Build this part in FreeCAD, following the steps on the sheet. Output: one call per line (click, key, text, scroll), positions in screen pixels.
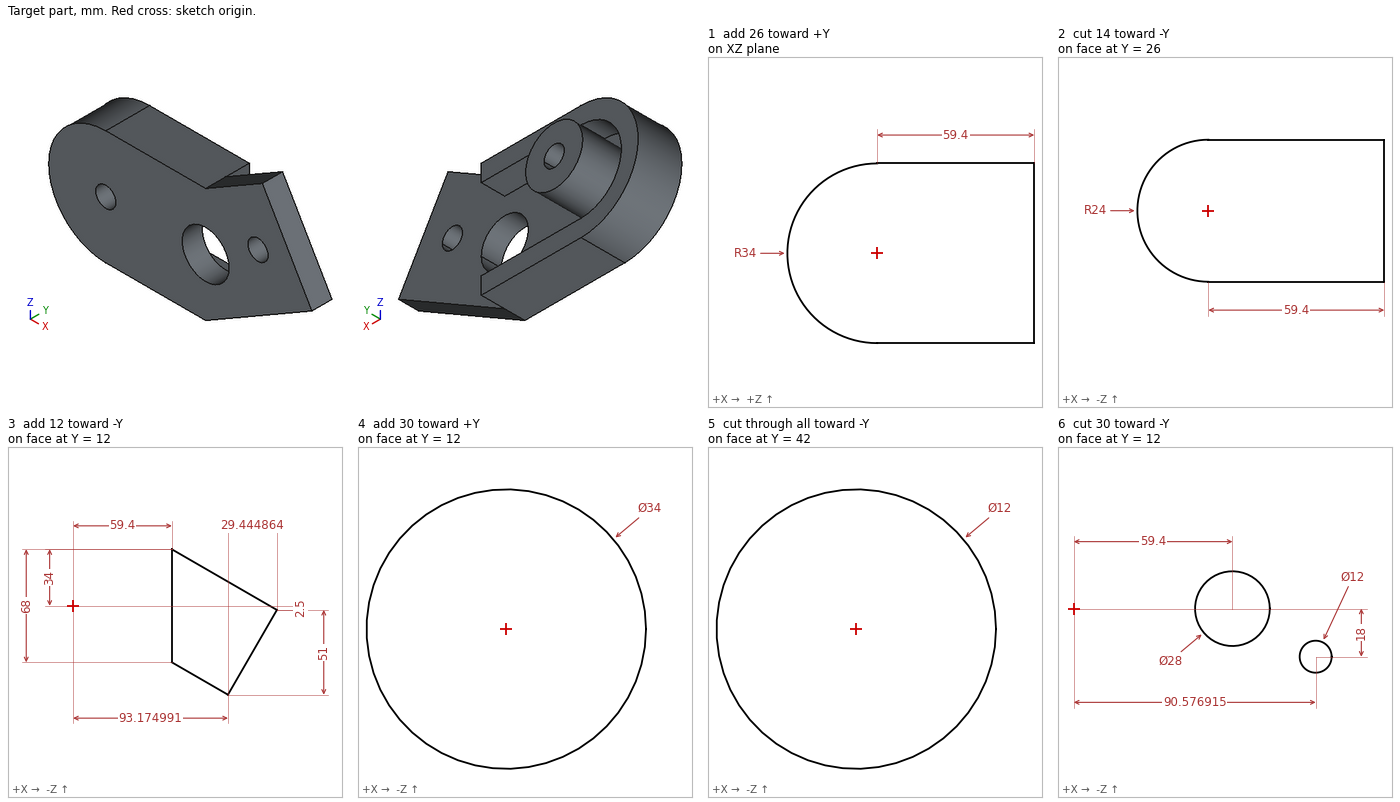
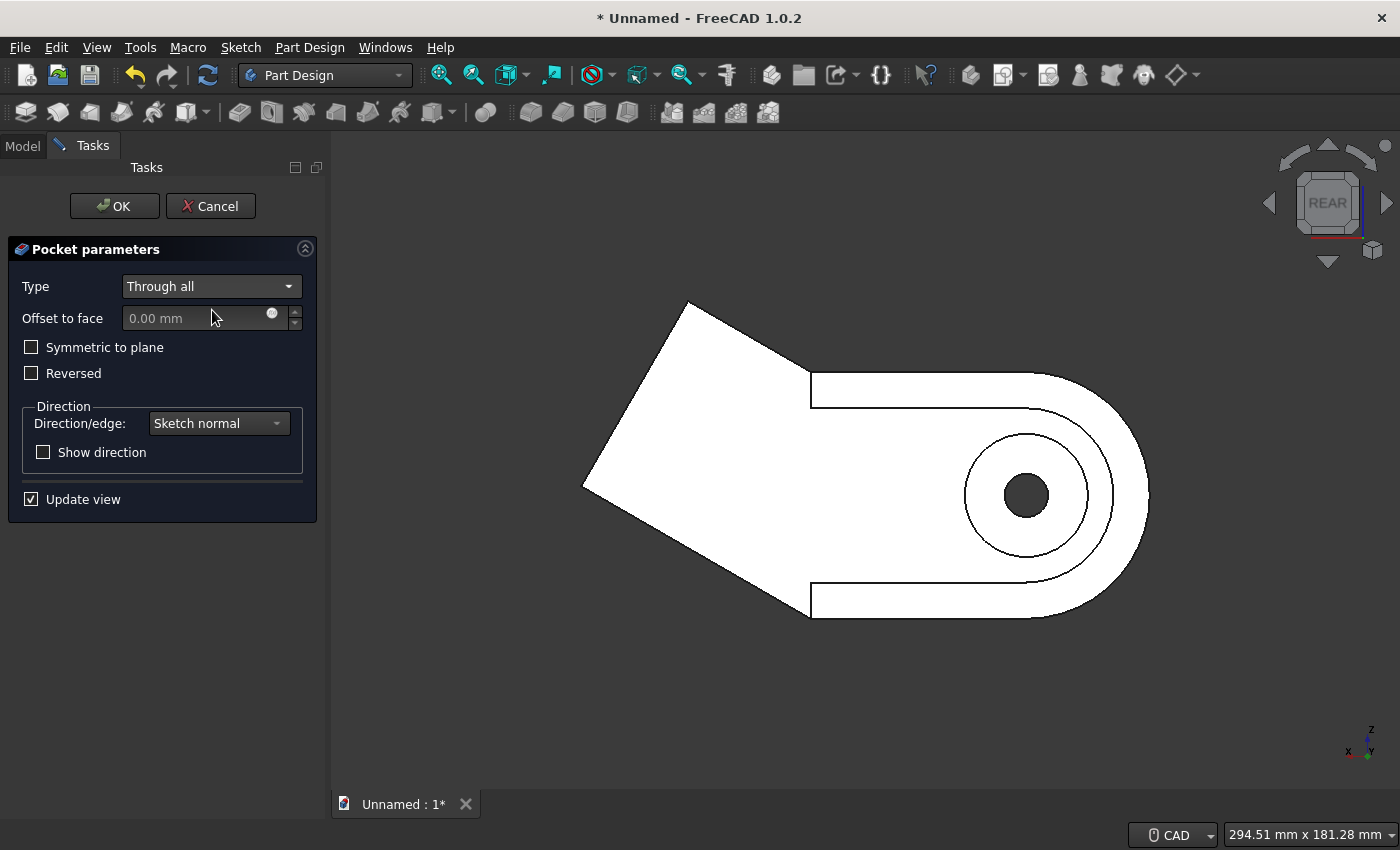
click(115, 206)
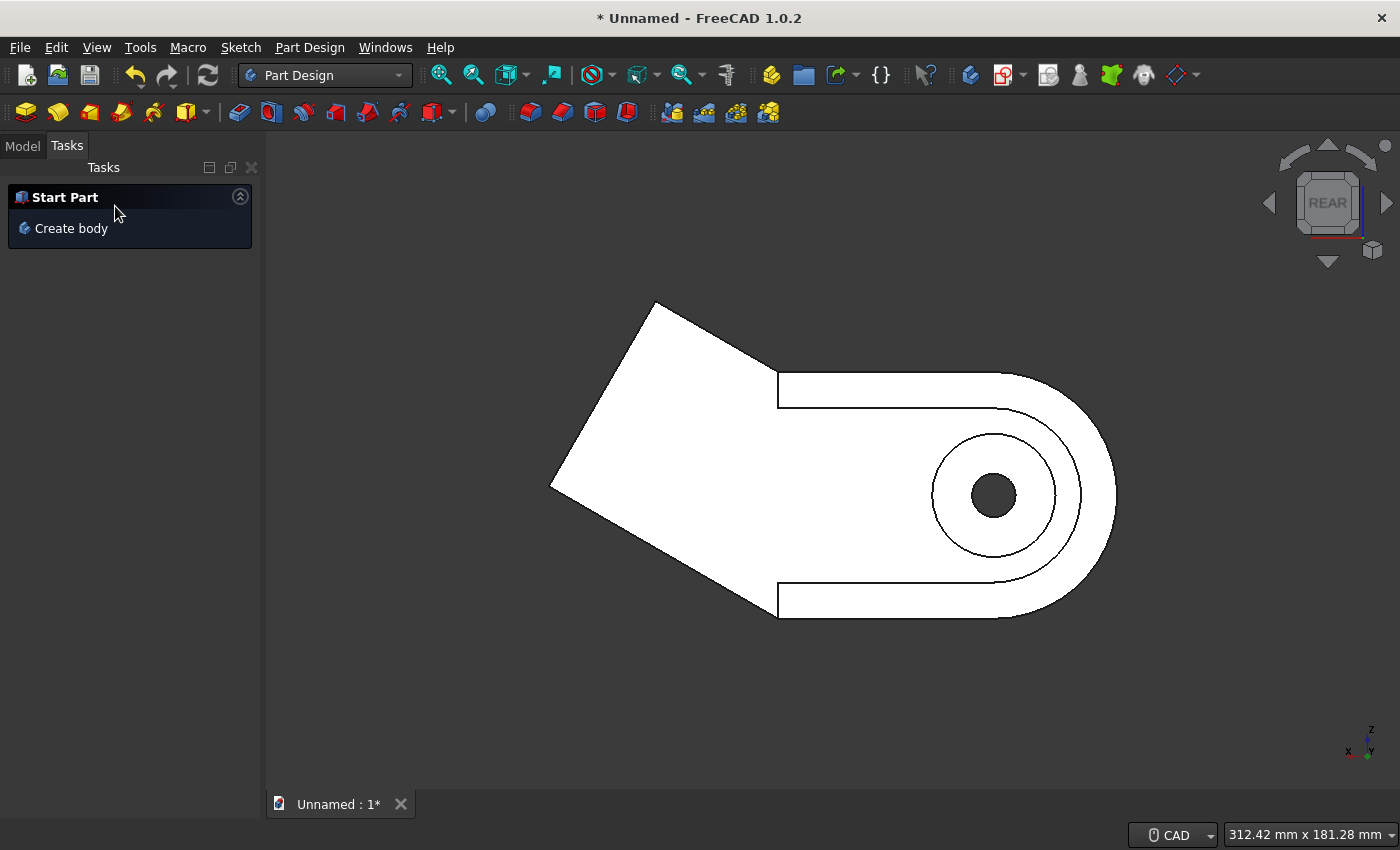
click(663, 459)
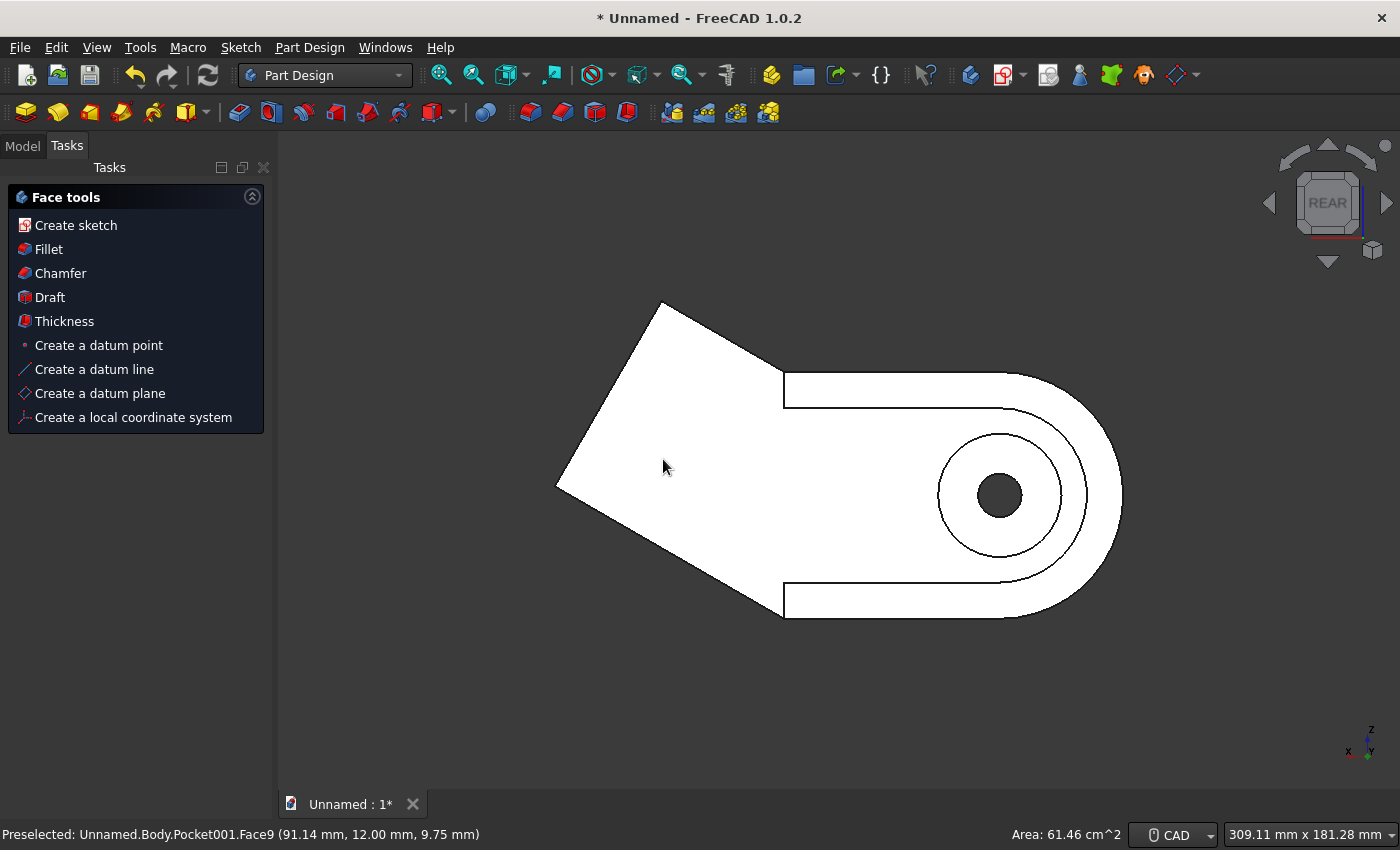
click(1004, 76)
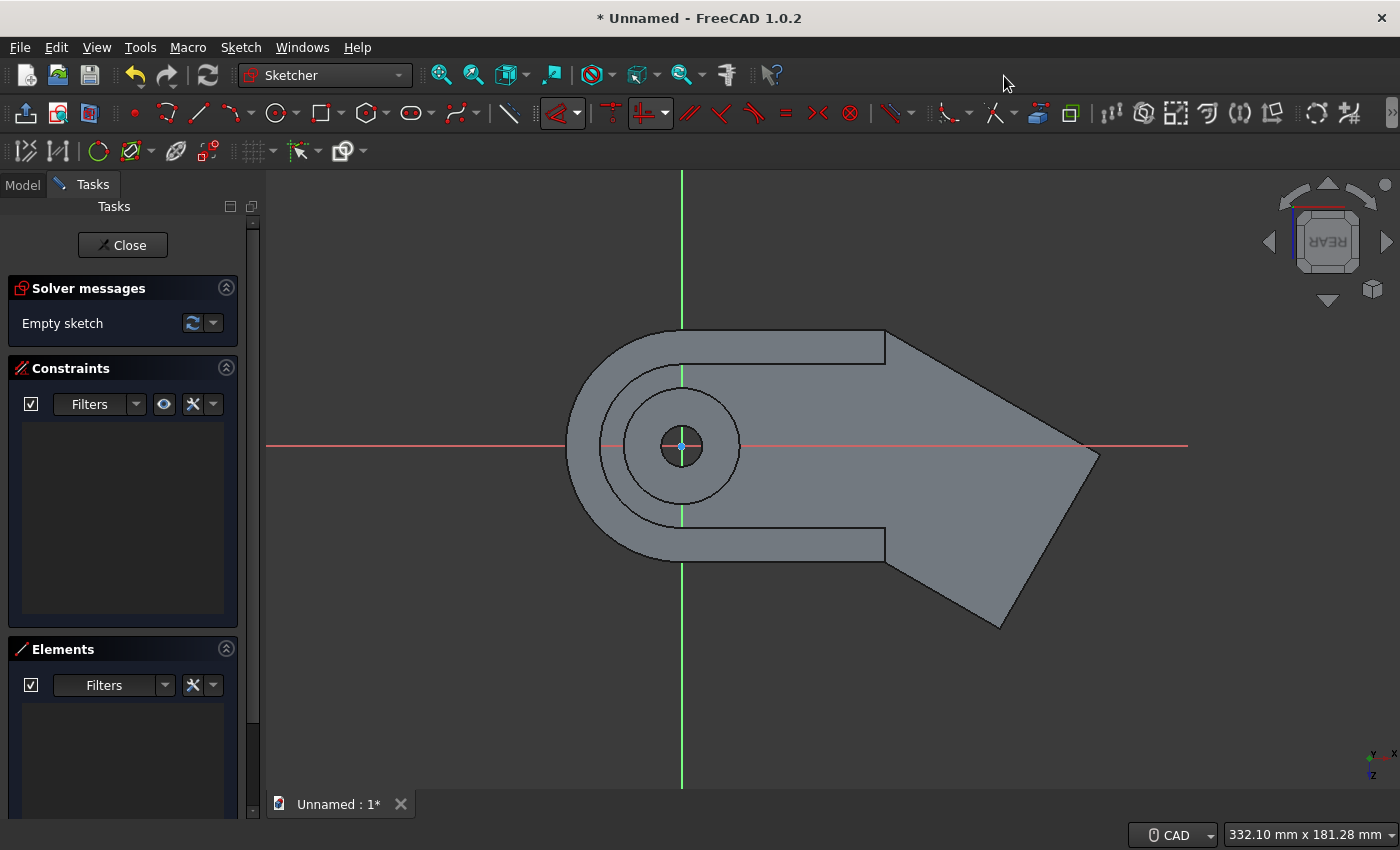
click(90, 114)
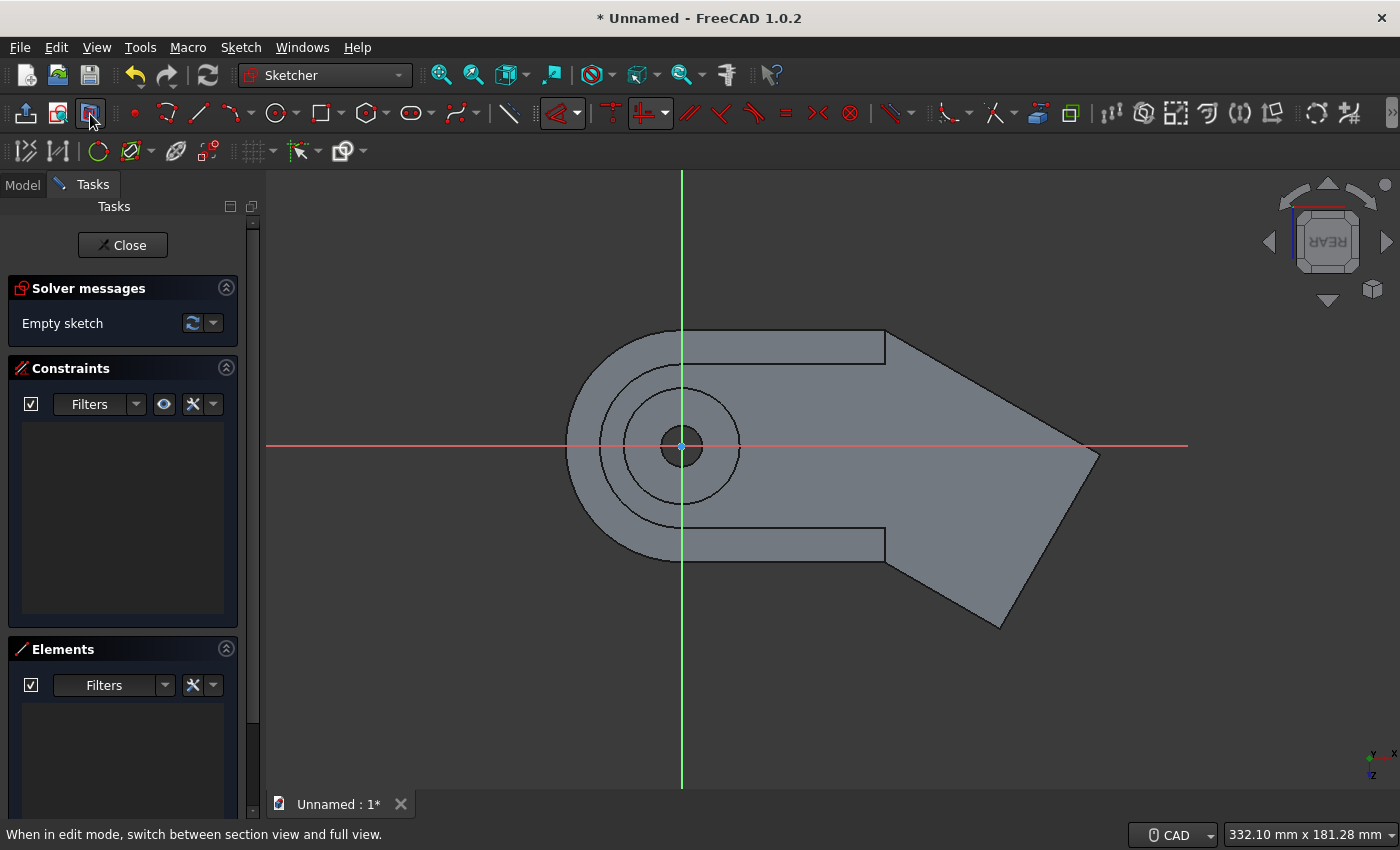
scroll(914, 450, up, 4)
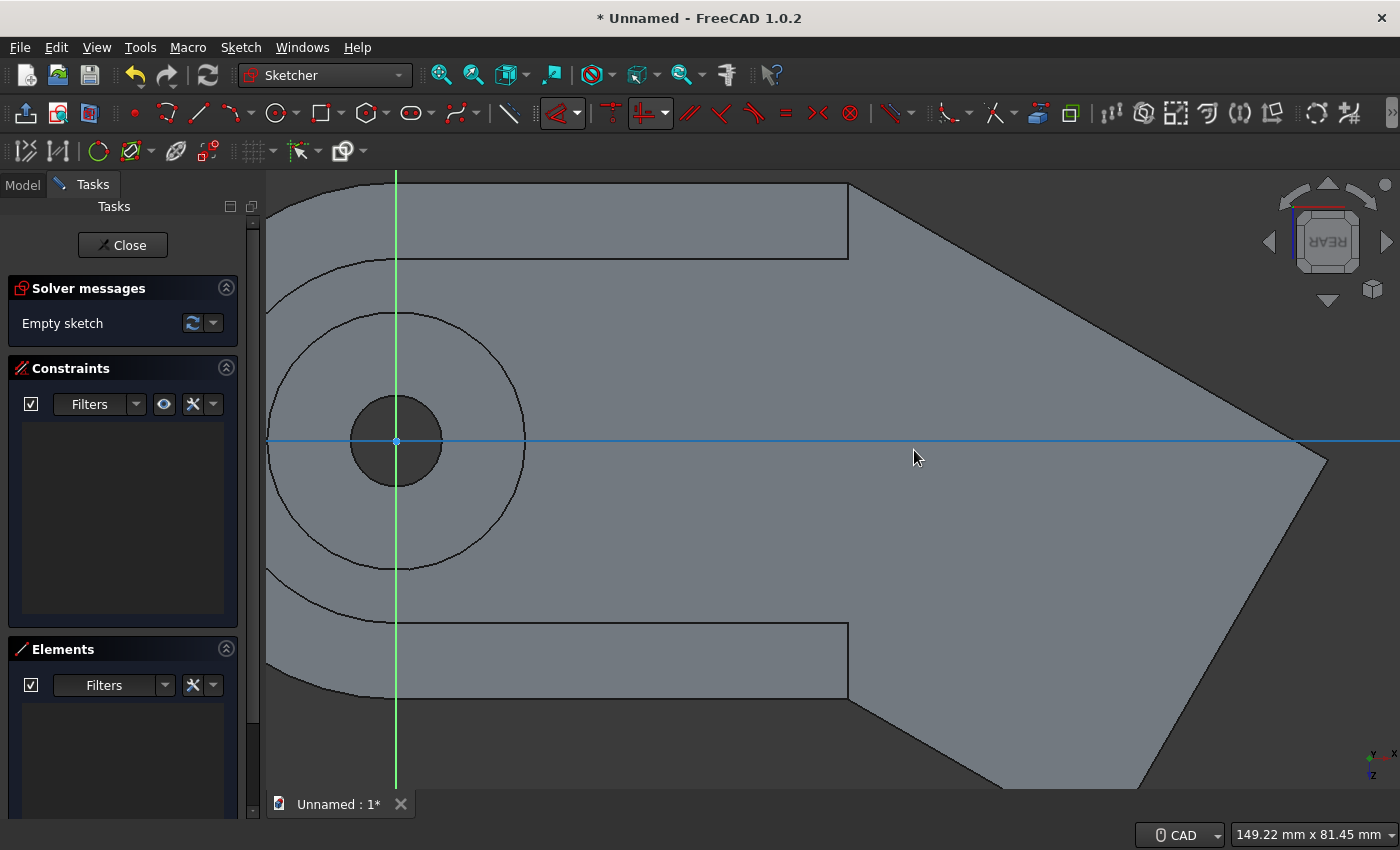
click(276, 114)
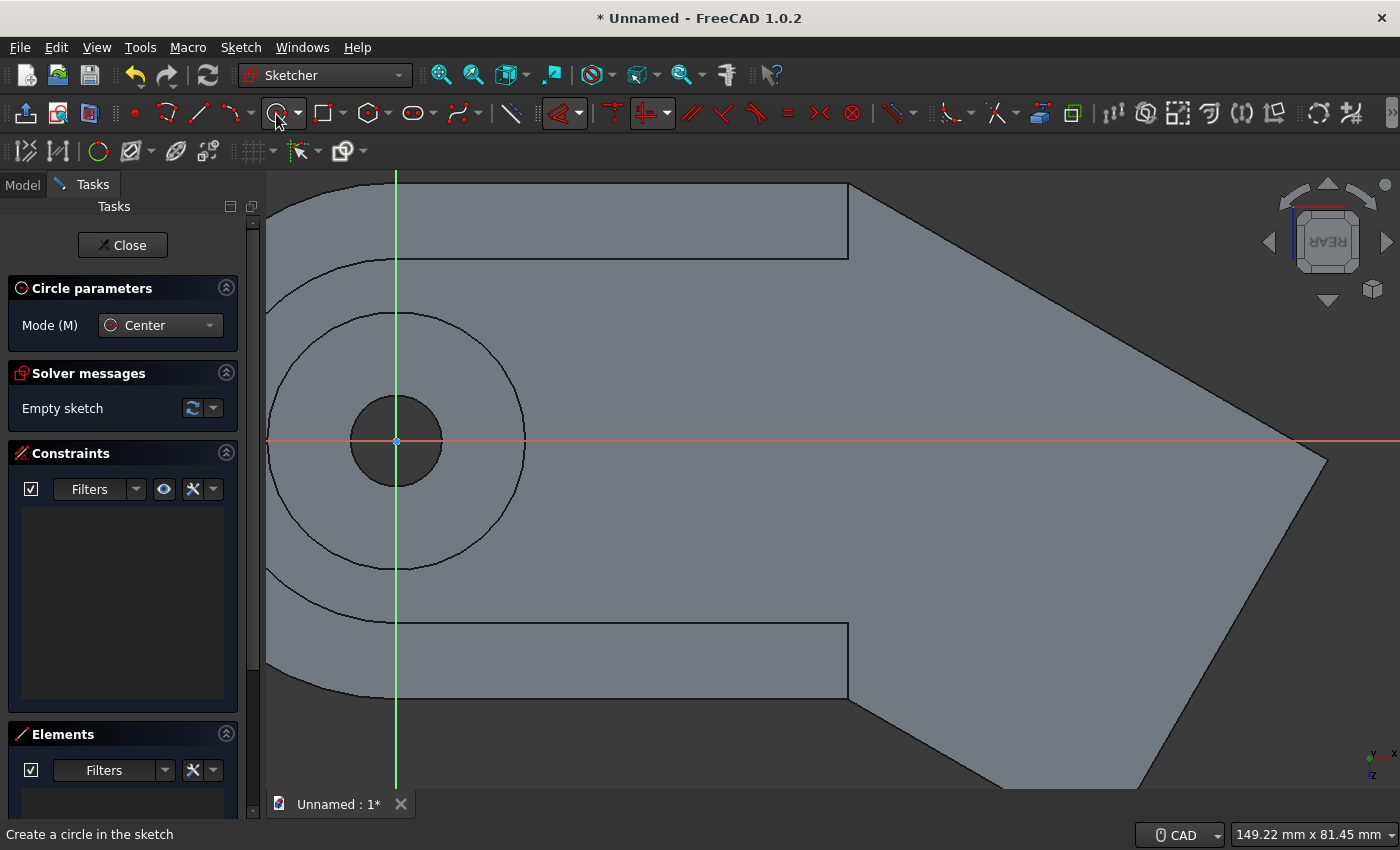
click(848, 441)
move(923, 366)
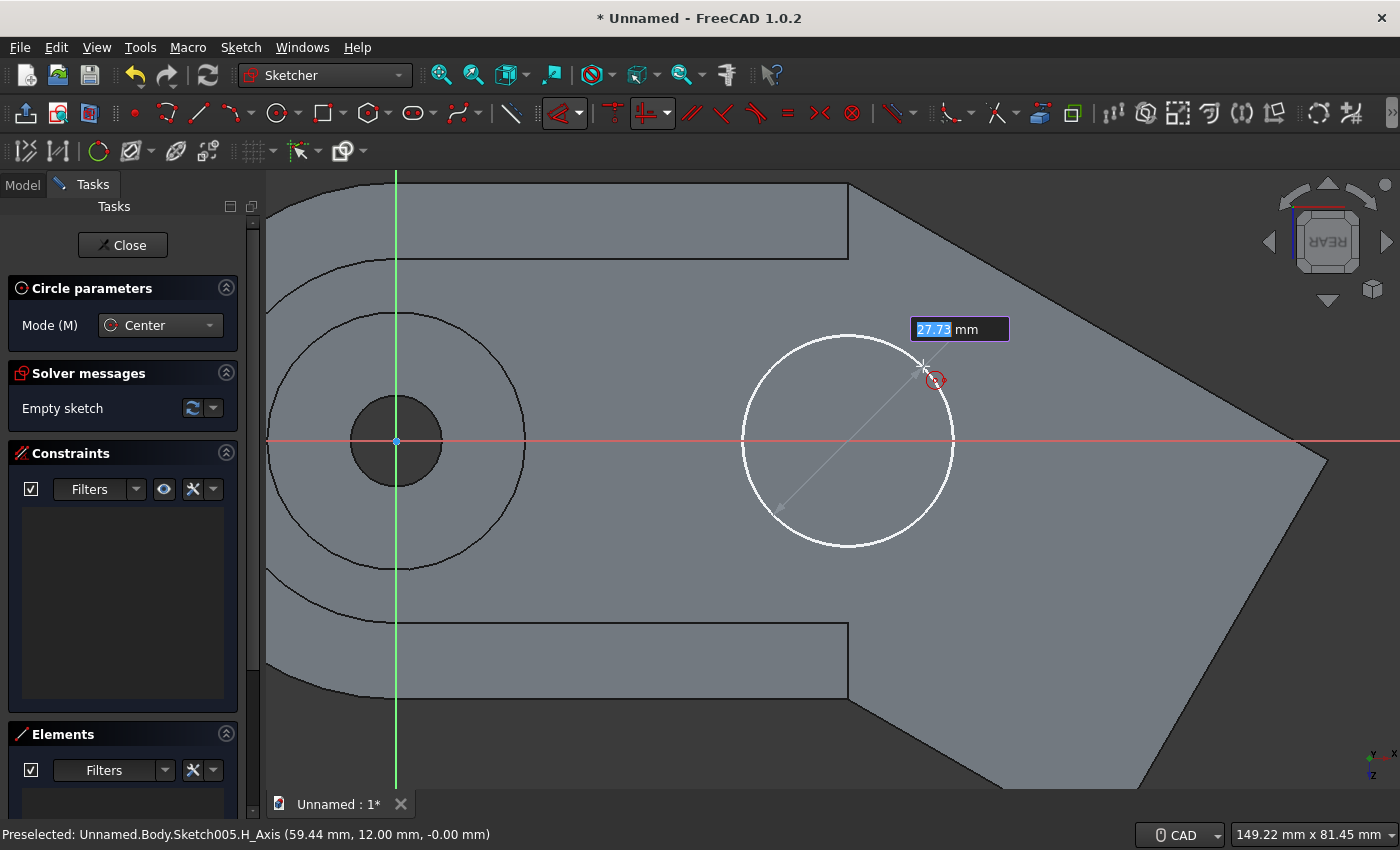
text(28)
key(Return)